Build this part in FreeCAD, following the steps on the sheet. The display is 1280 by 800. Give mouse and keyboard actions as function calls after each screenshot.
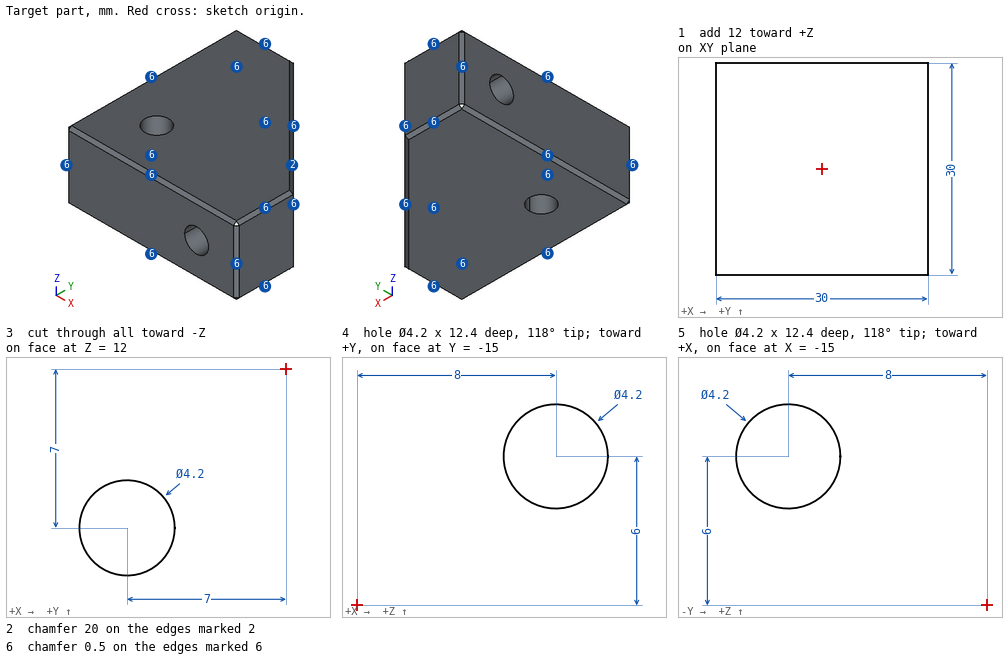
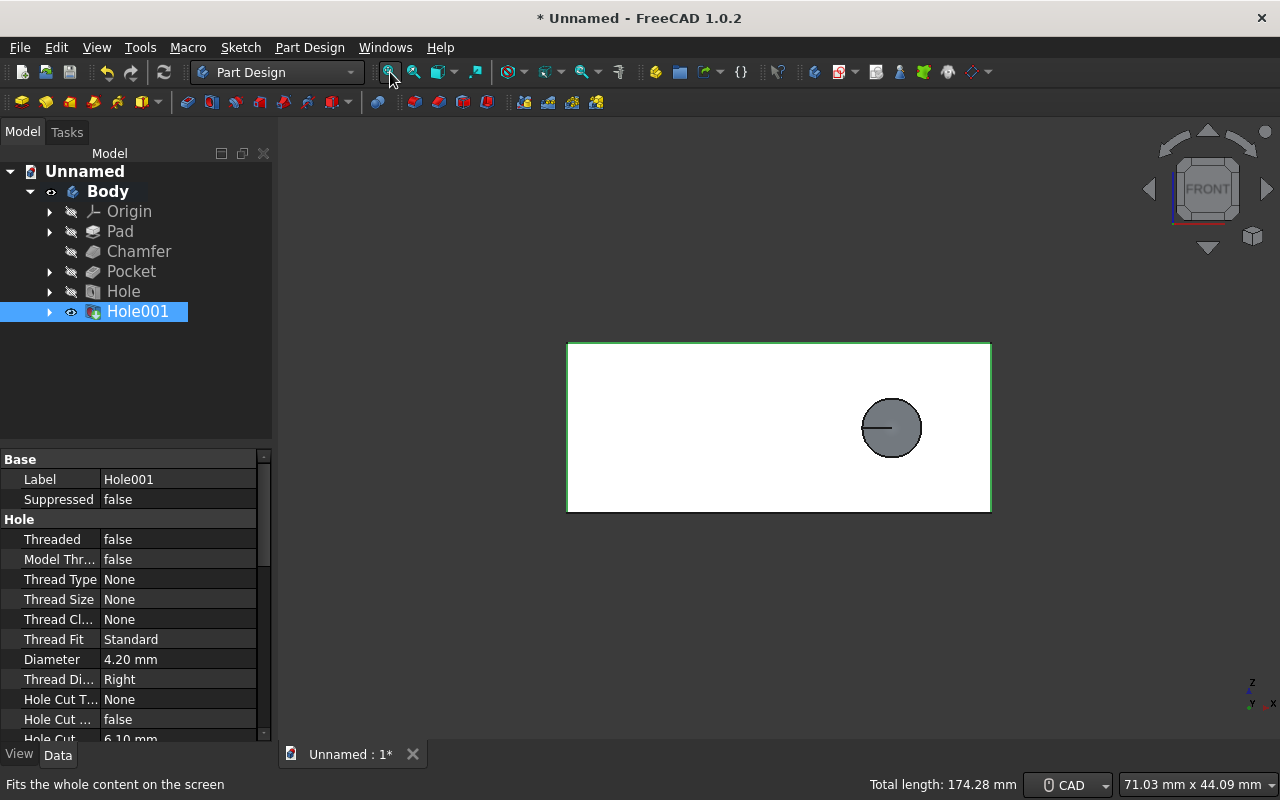
click(779, 512, ctrl)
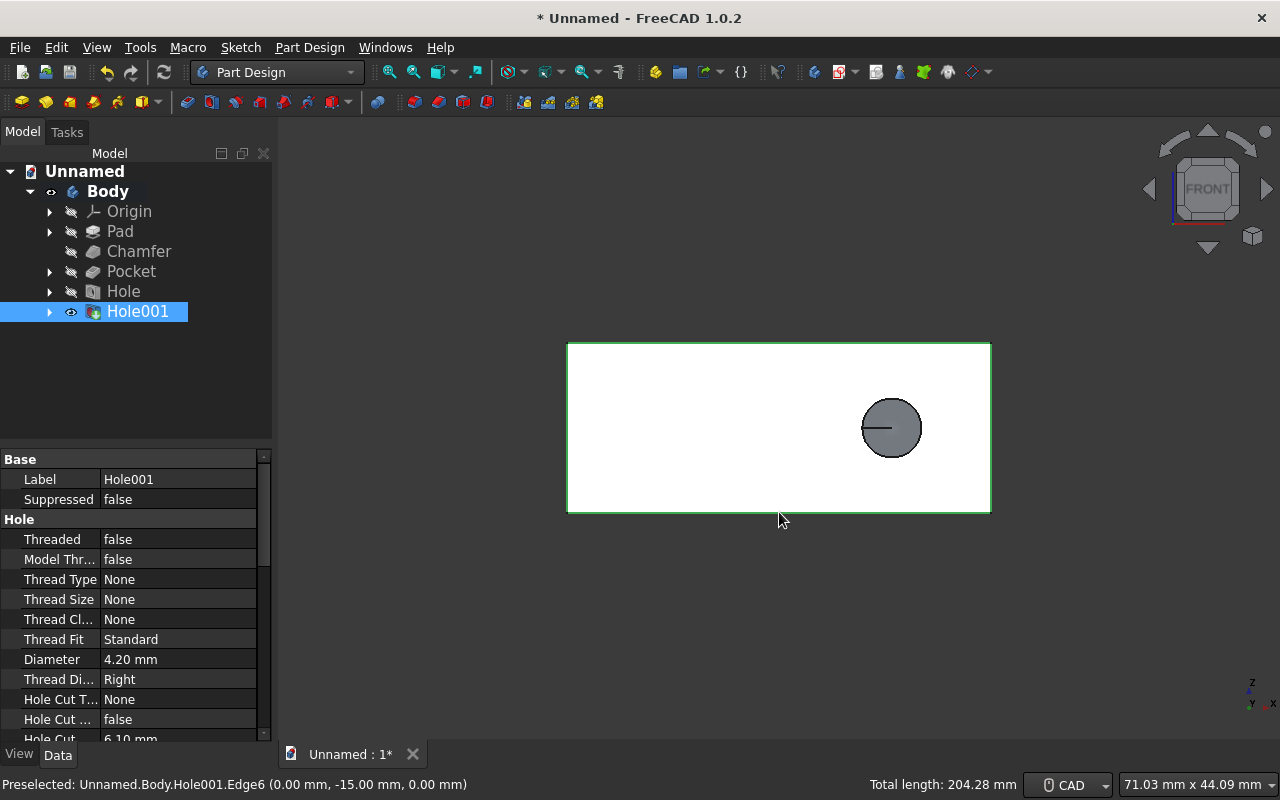
key(3)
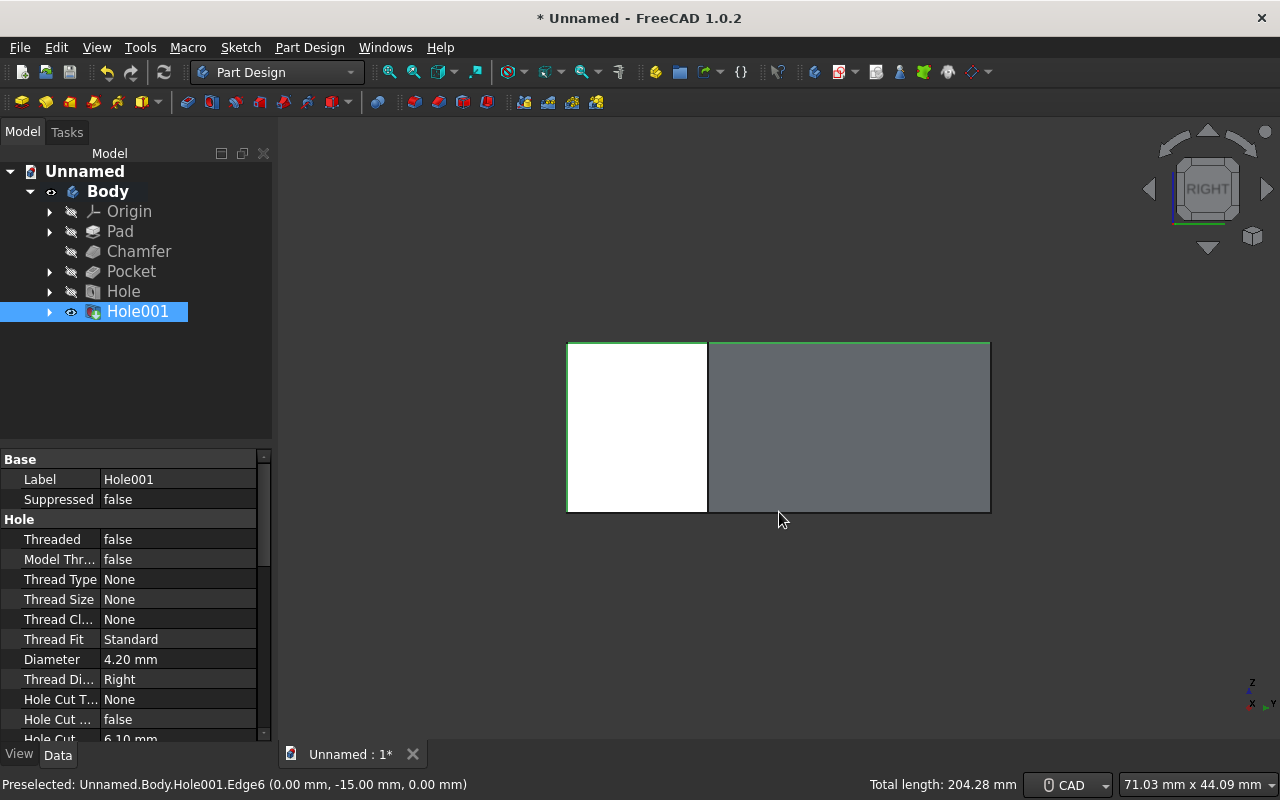
key(v)
key(f)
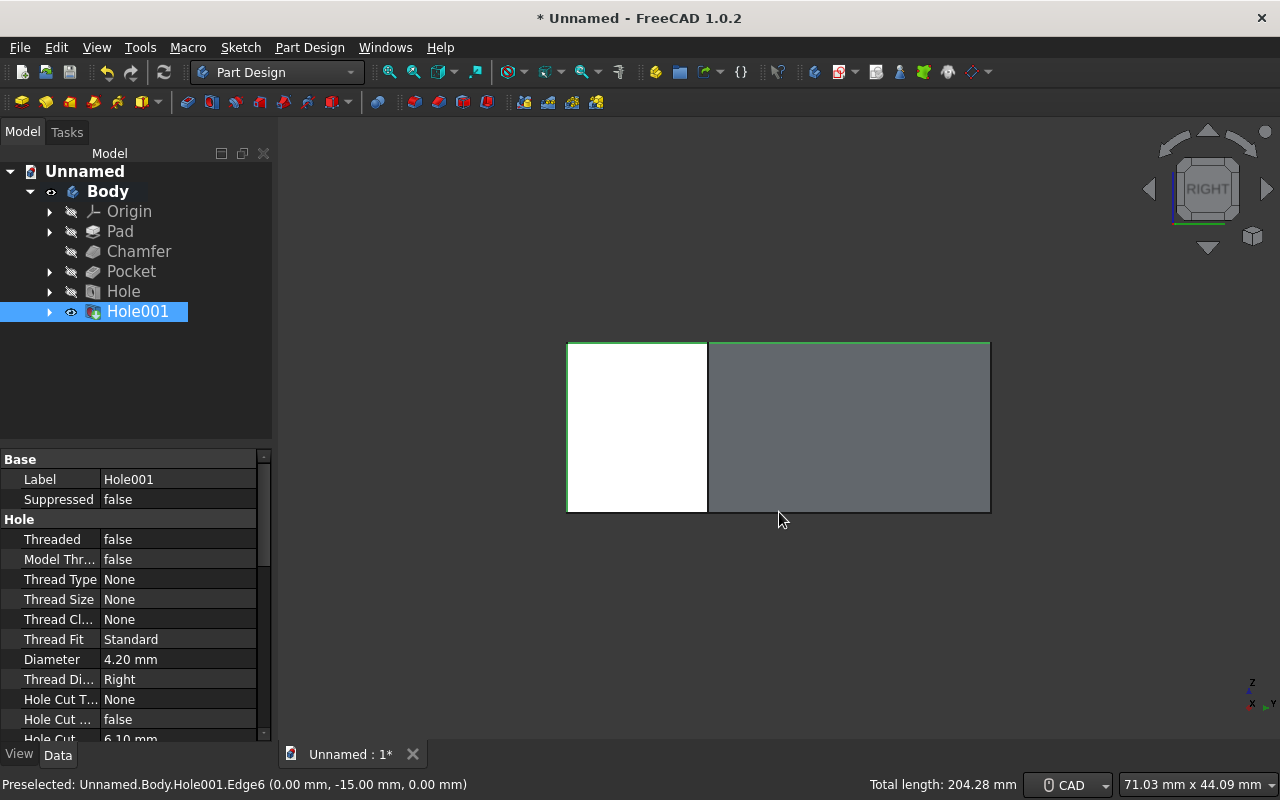
click(850, 512, ctrl)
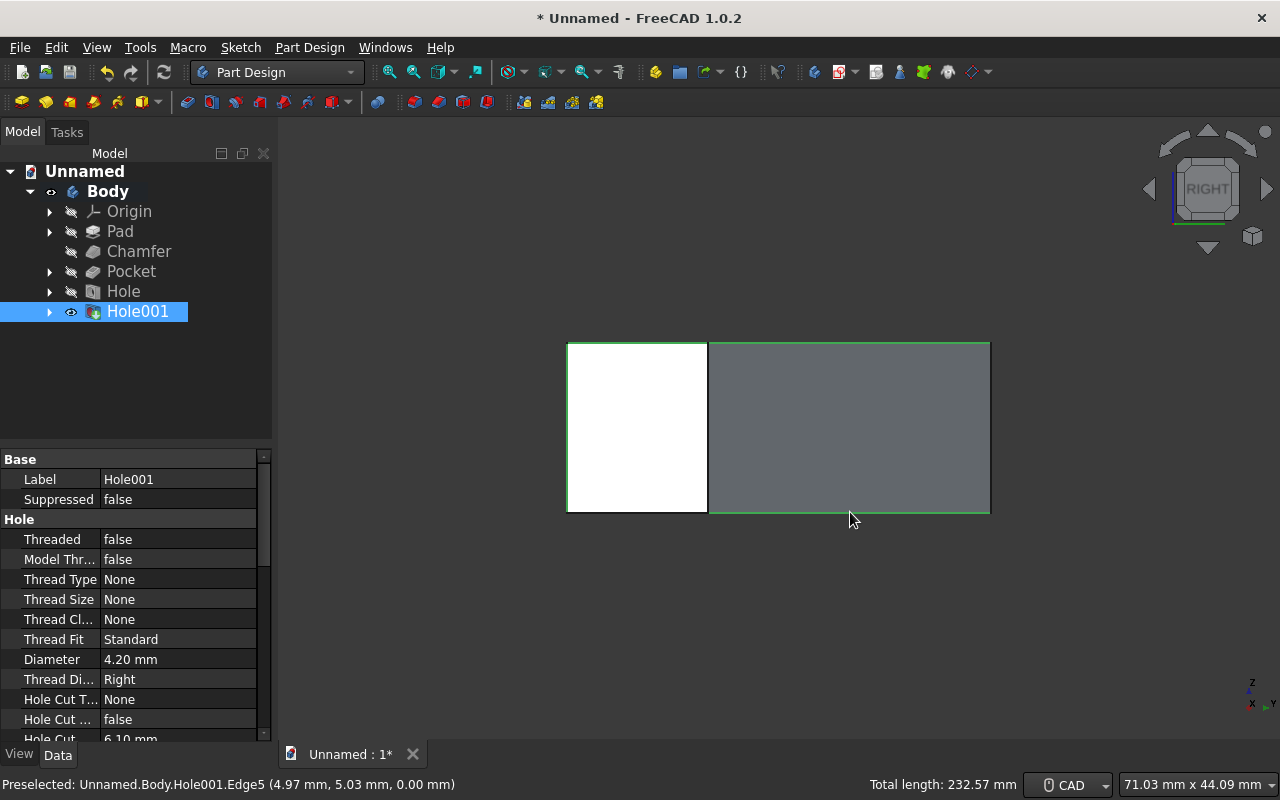
click(638, 512, ctrl)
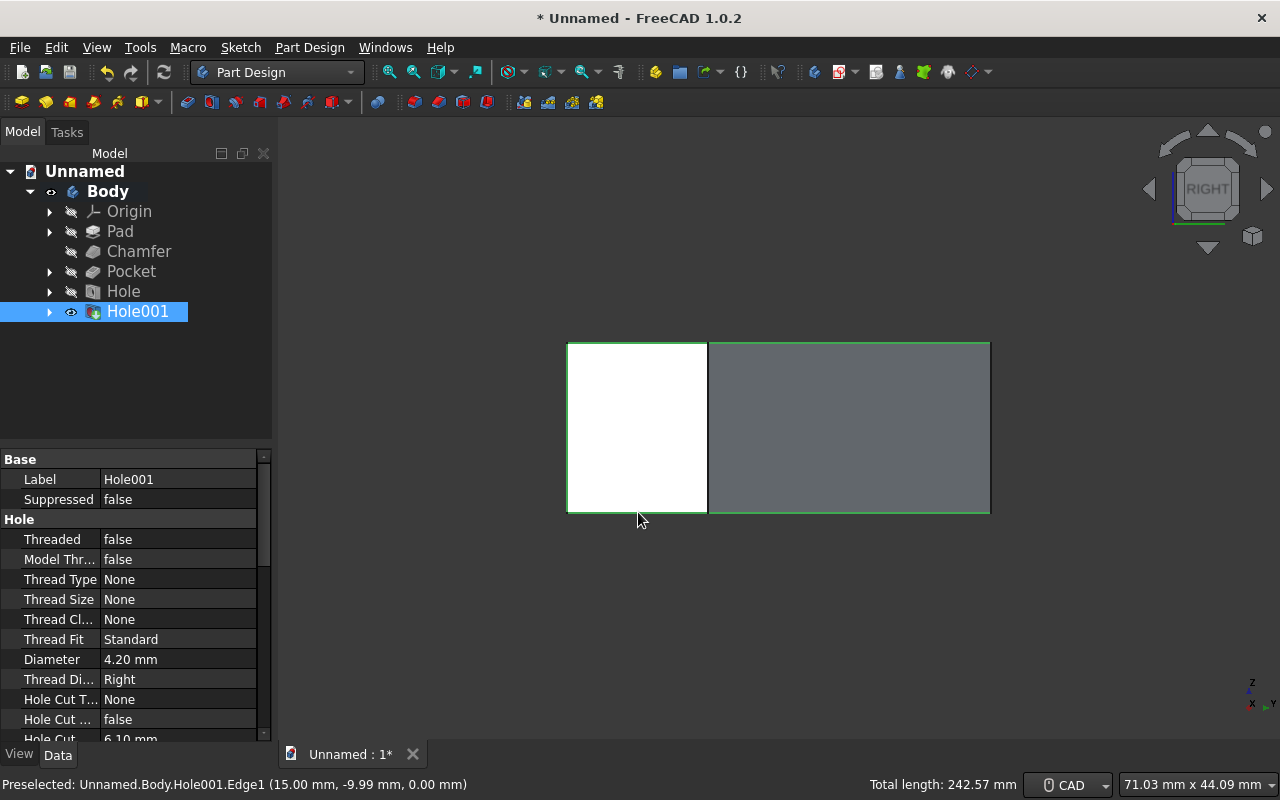
key(5)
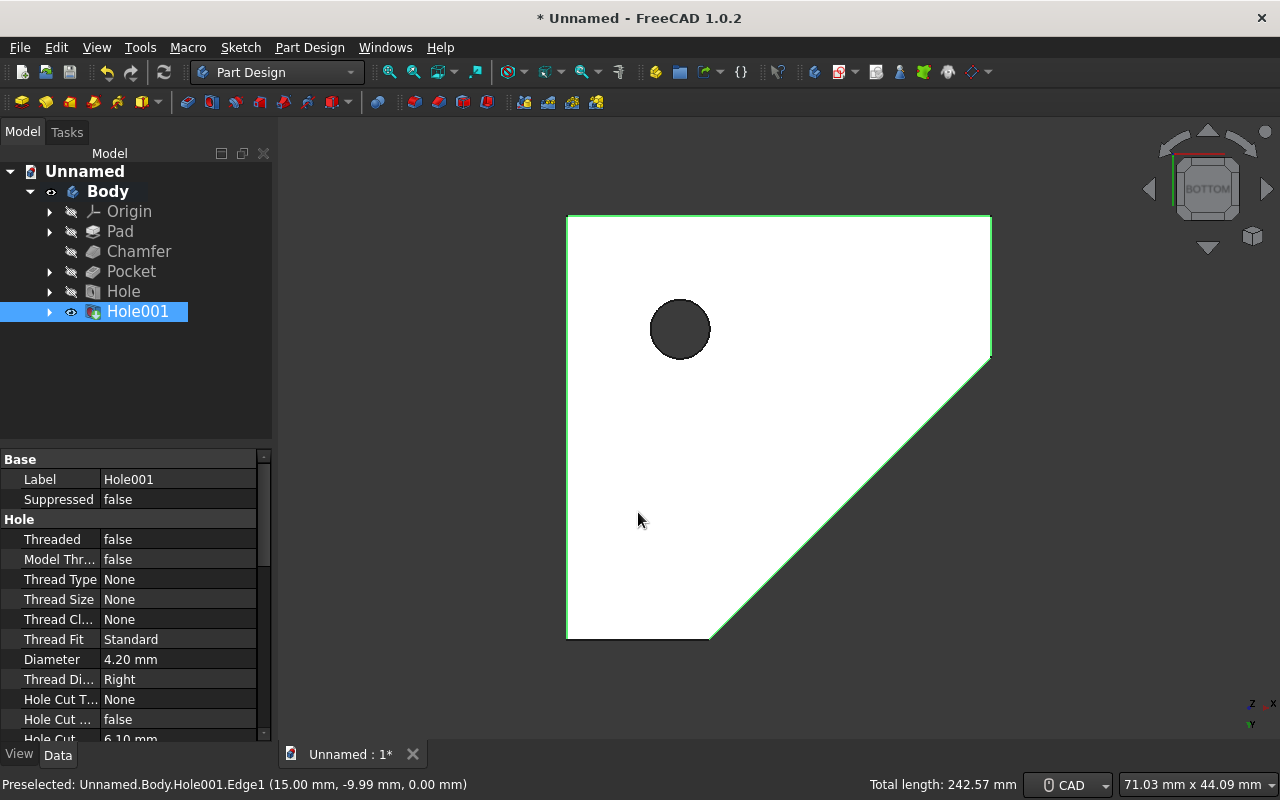
click(638, 639, ctrl)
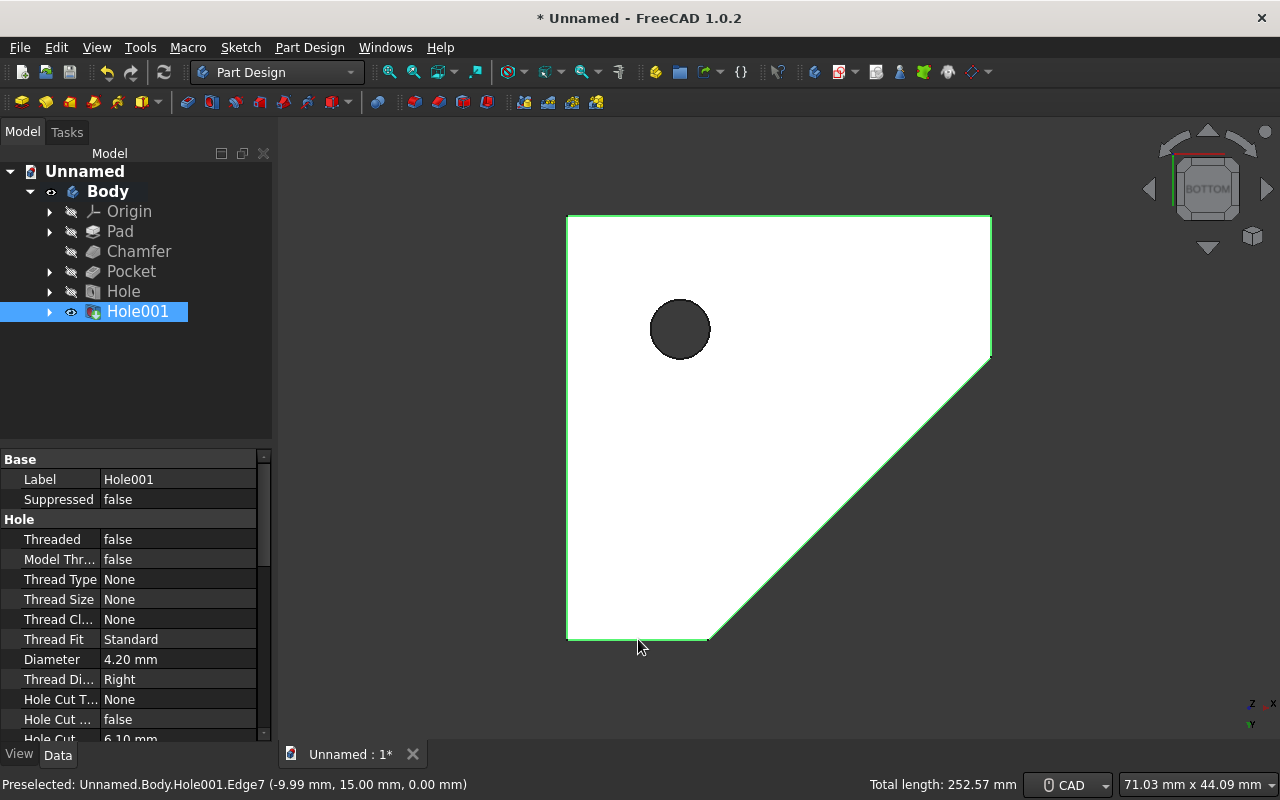
click(440, 102)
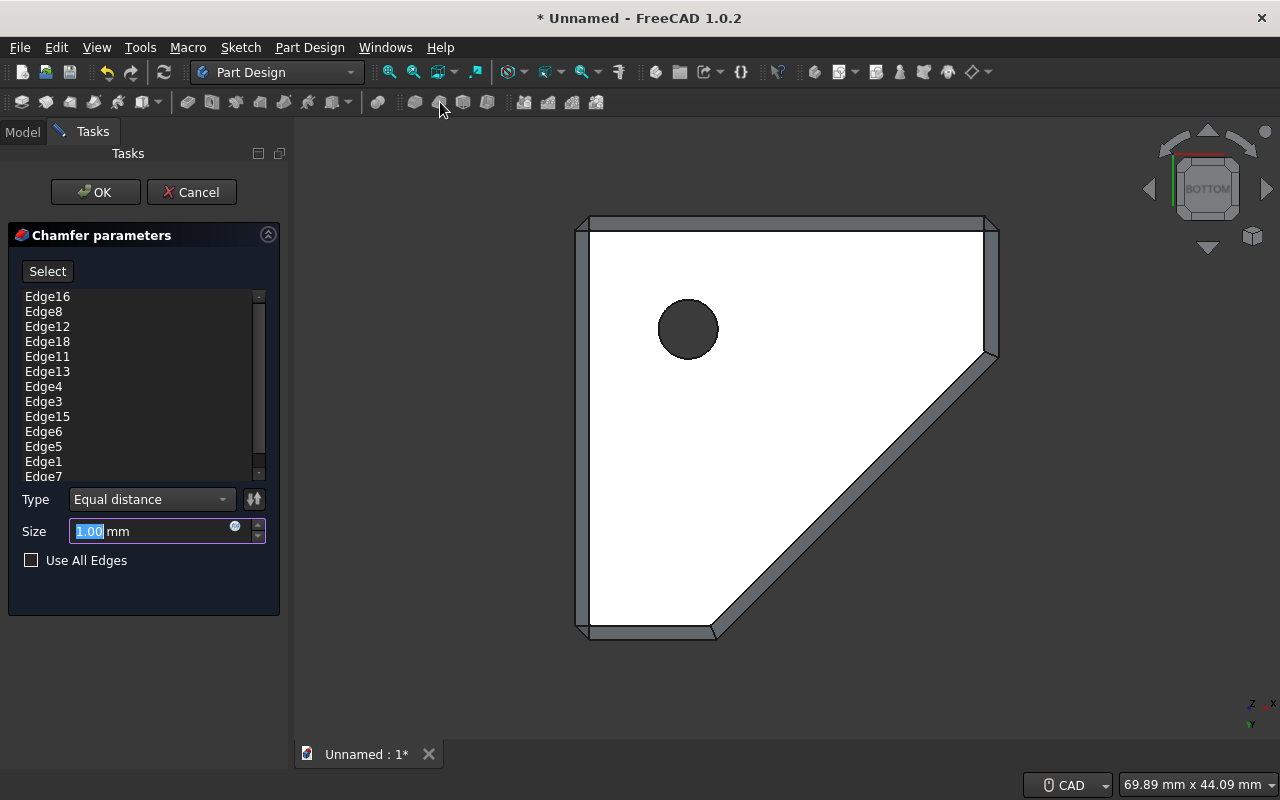
text(0.5)
key(Tab)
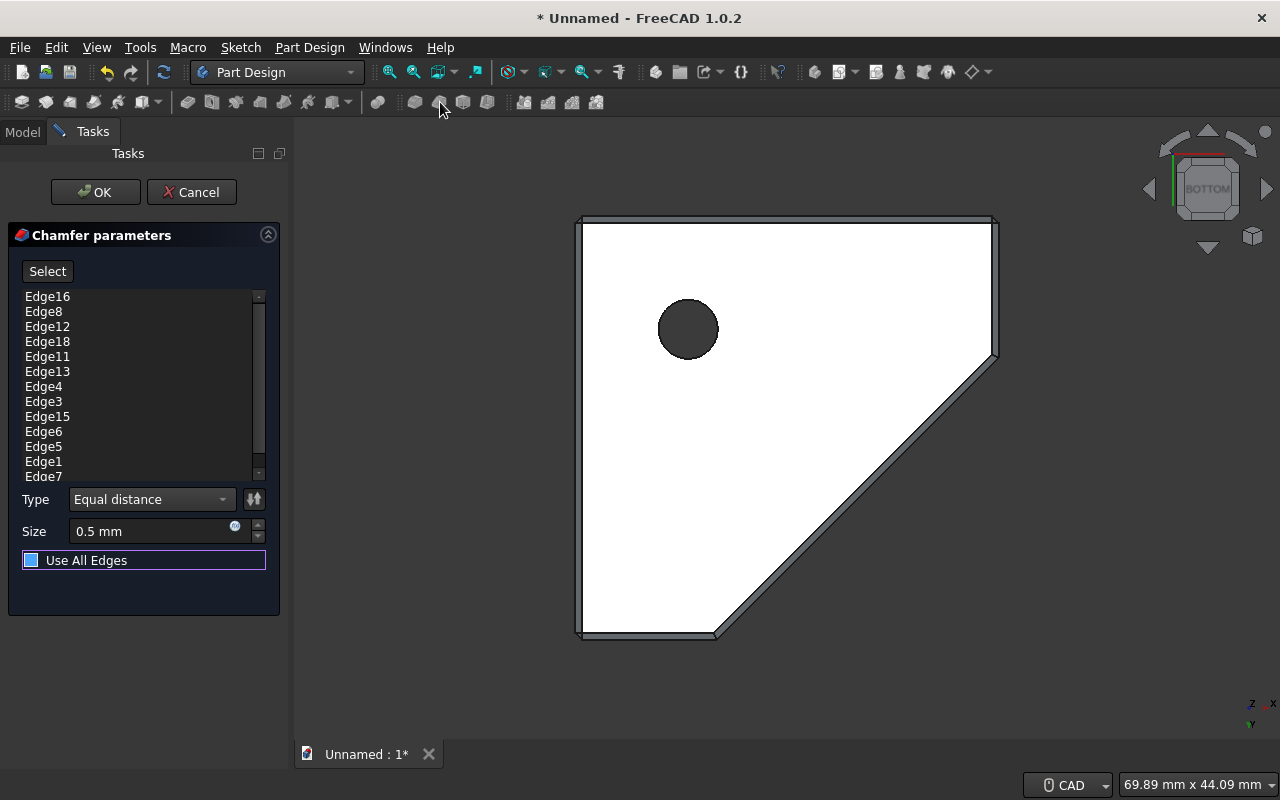
click(96, 192)